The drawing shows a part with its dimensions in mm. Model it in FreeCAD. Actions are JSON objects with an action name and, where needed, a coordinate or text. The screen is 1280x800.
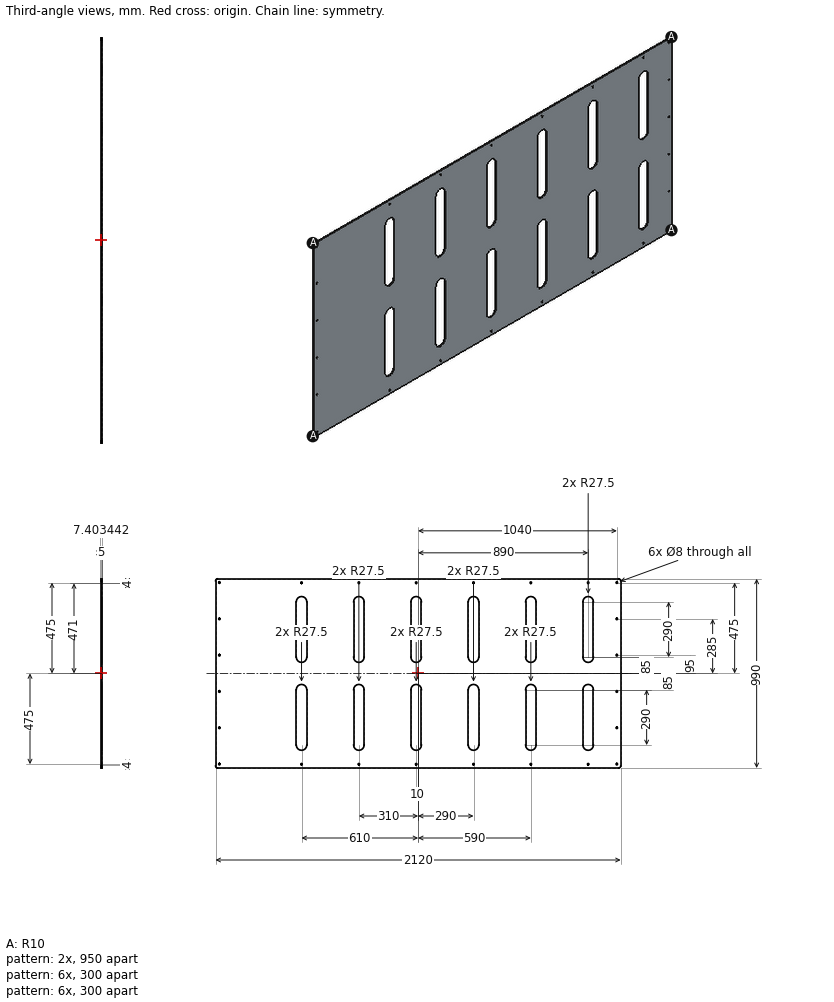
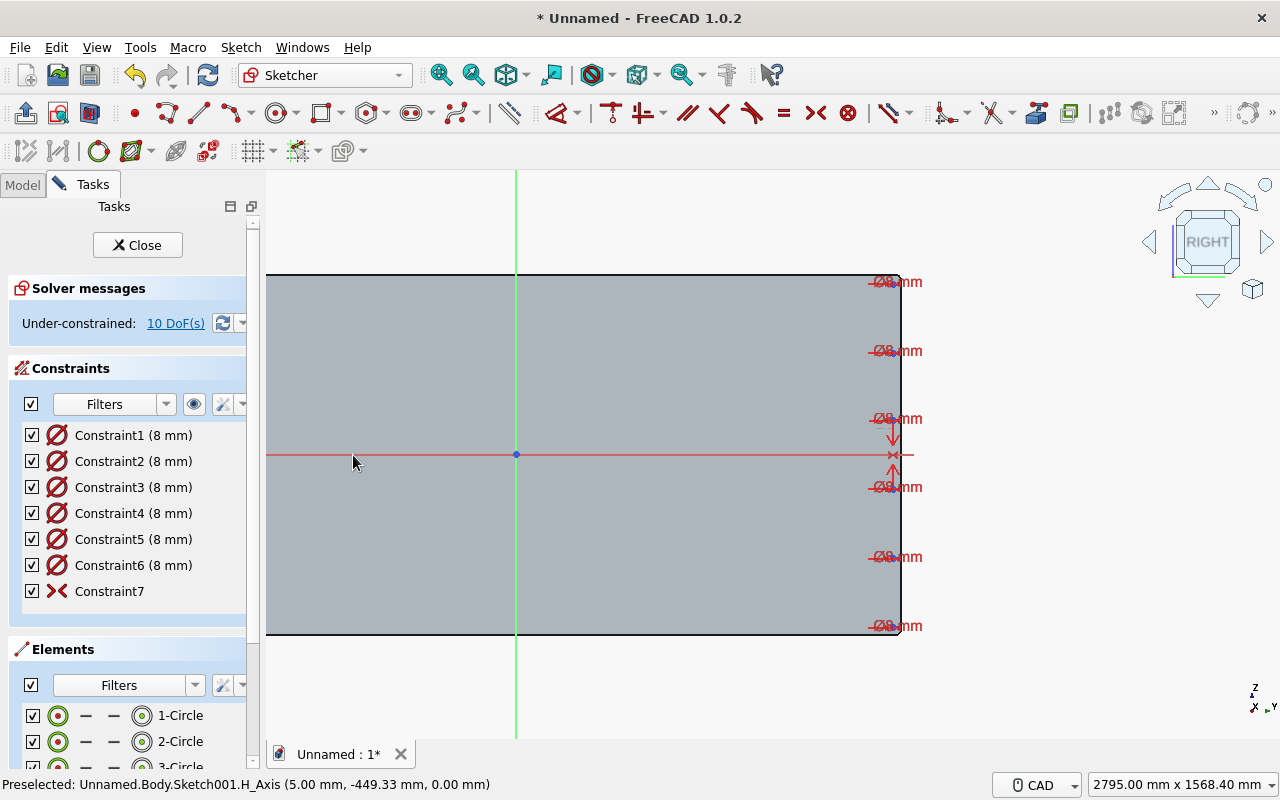
{"action": "left_click", "coordinate": [893, 353]}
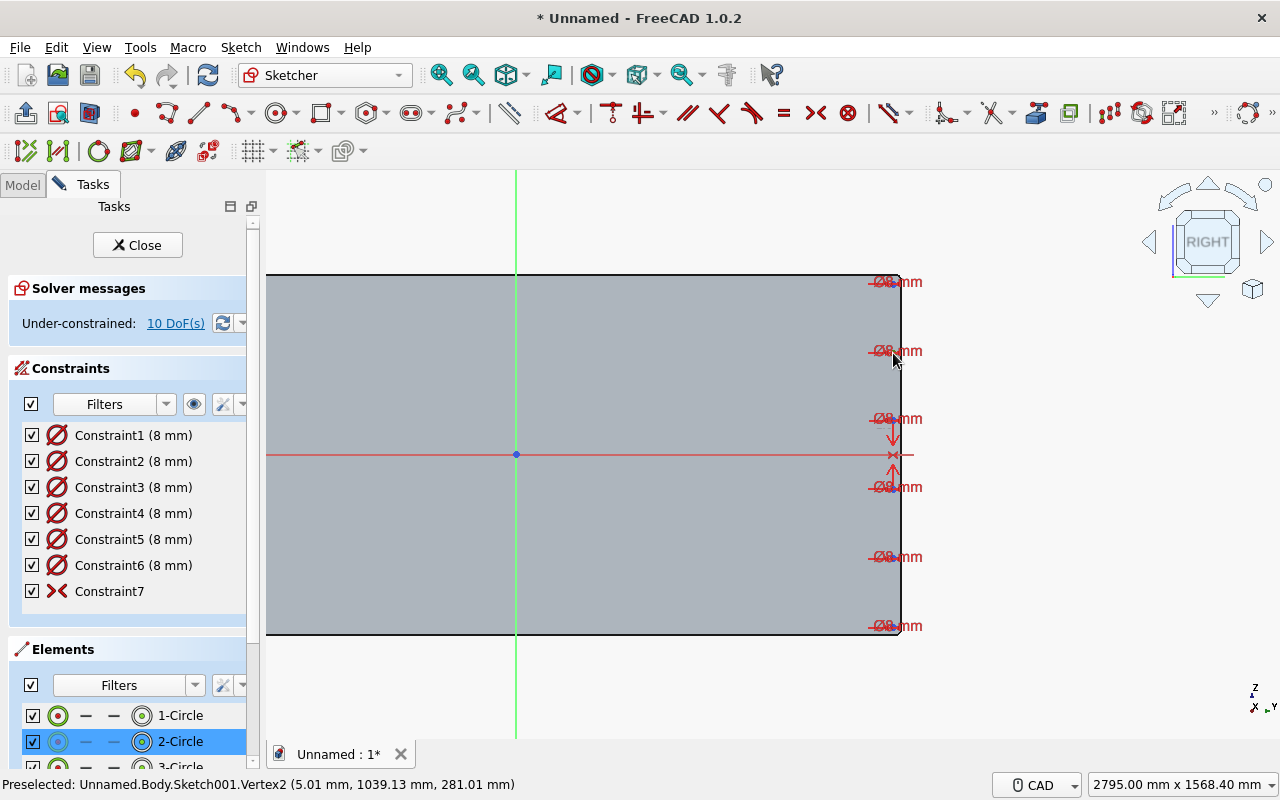
{"action": "left_click", "coordinate": [893, 559]}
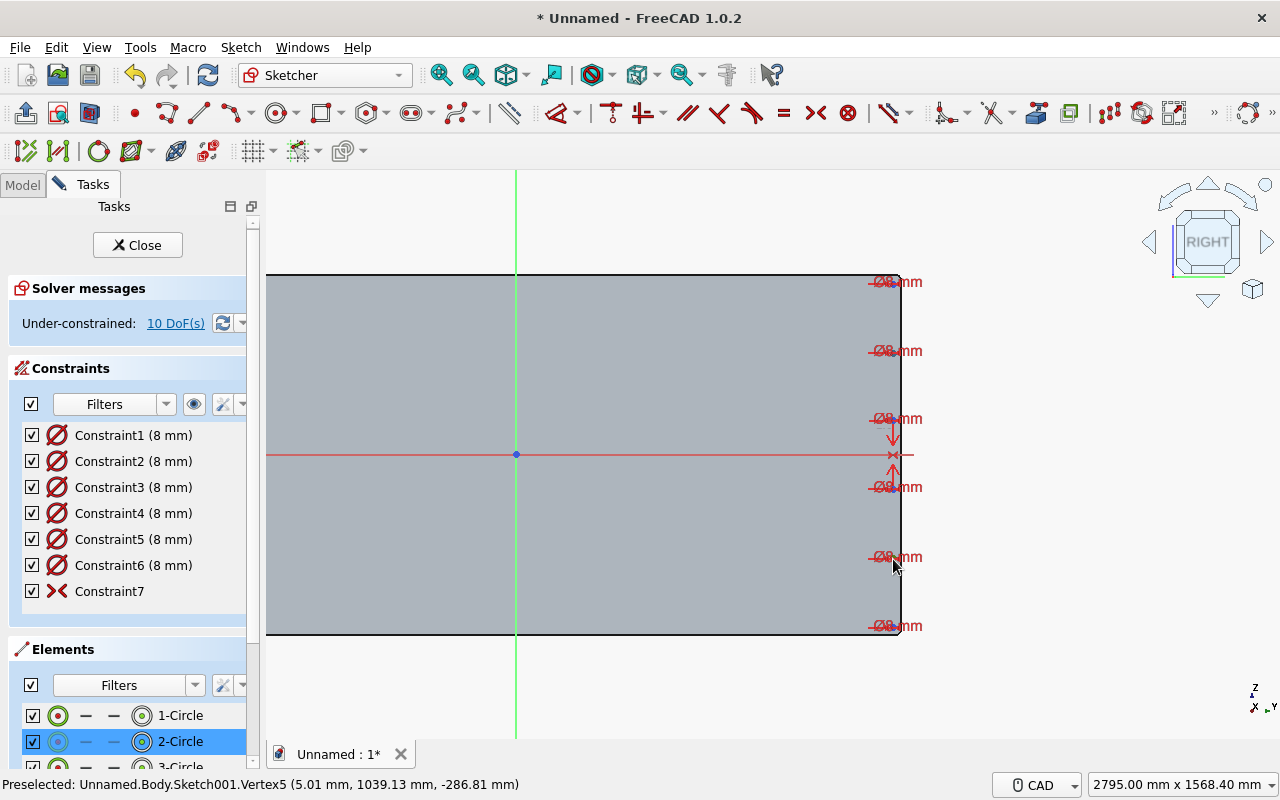
{"action": "left_click", "coordinate": [353, 455]}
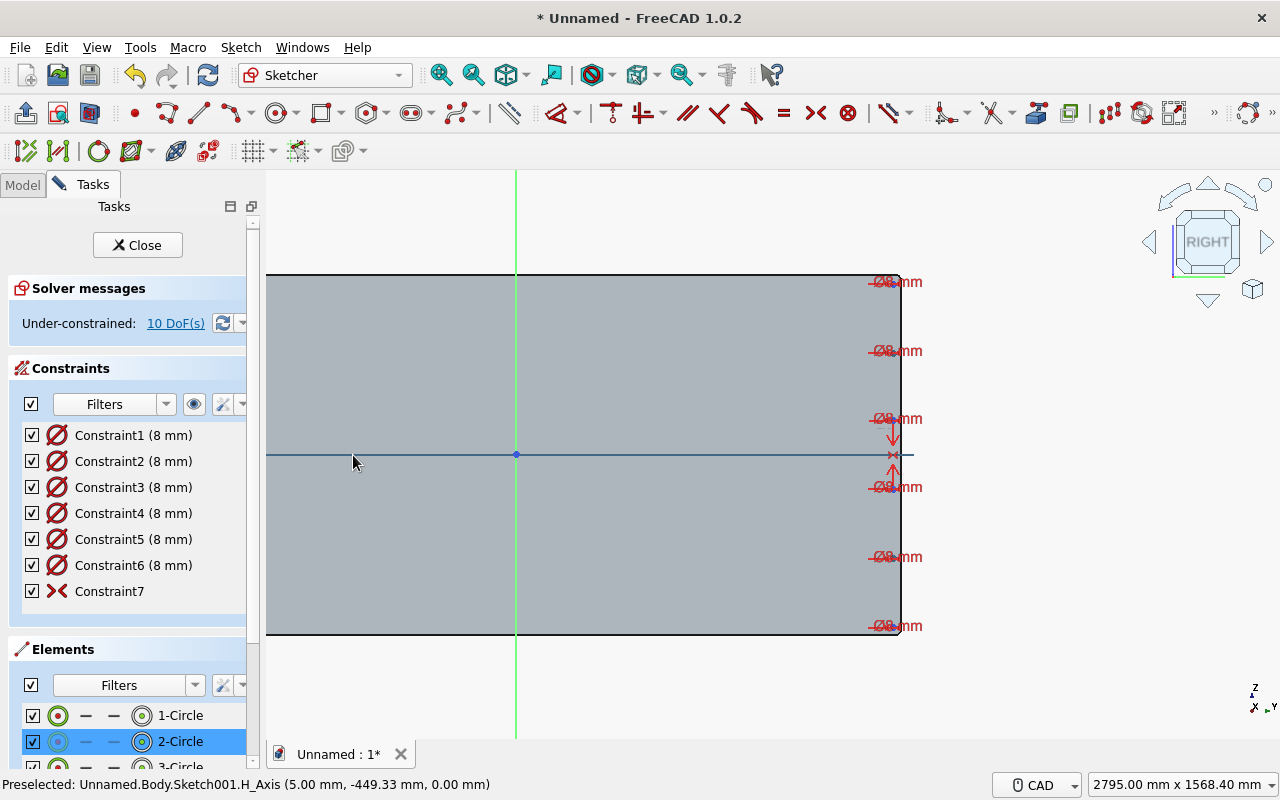
{"action": "left_click", "coordinate": [816, 114]}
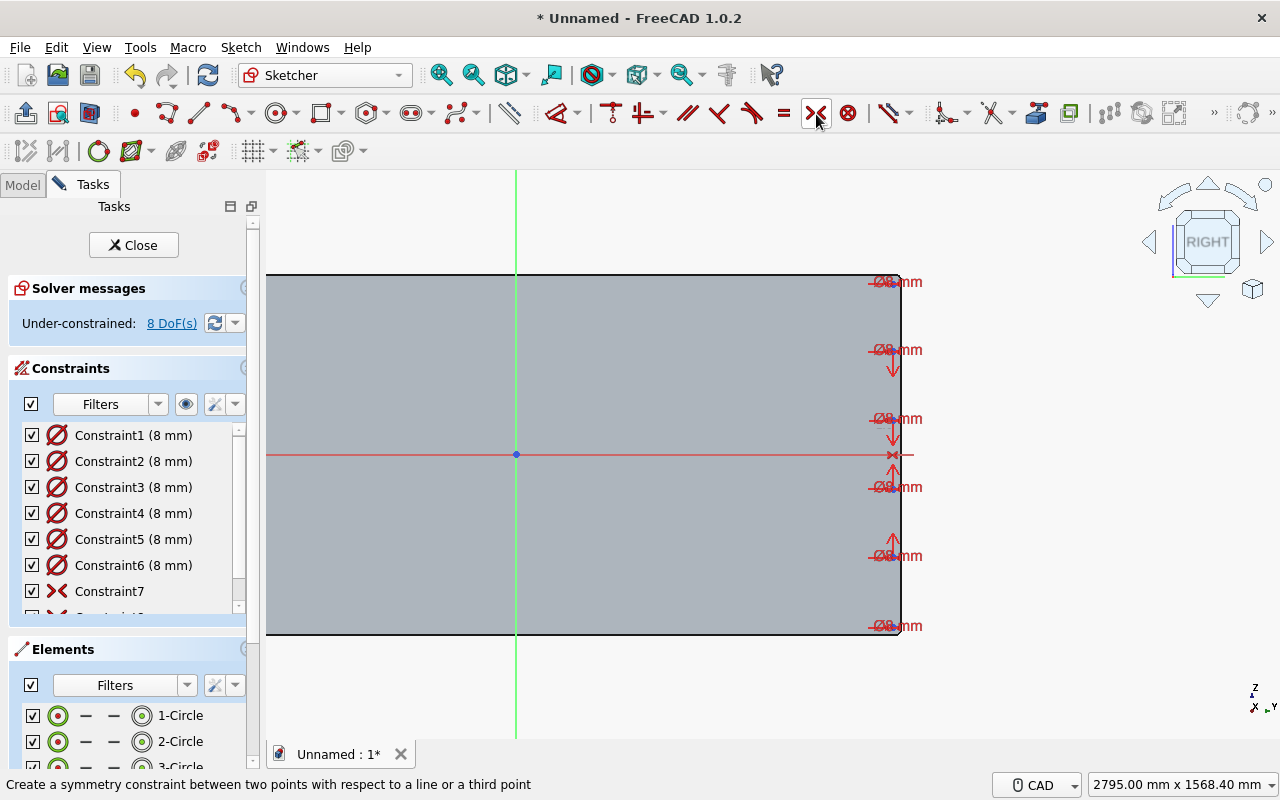
{"action": "left_click", "coordinate": [893, 284]}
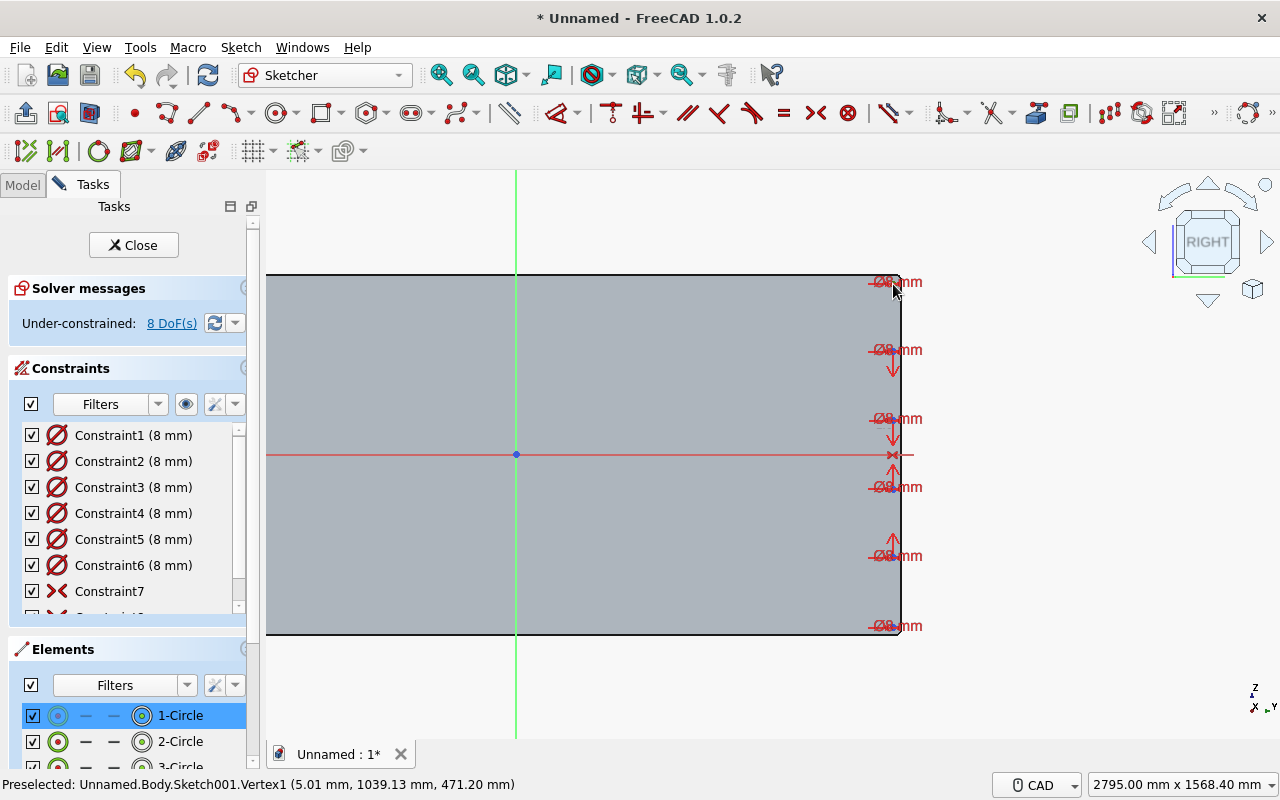
{"action": "left_click", "coordinate": [893, 628]}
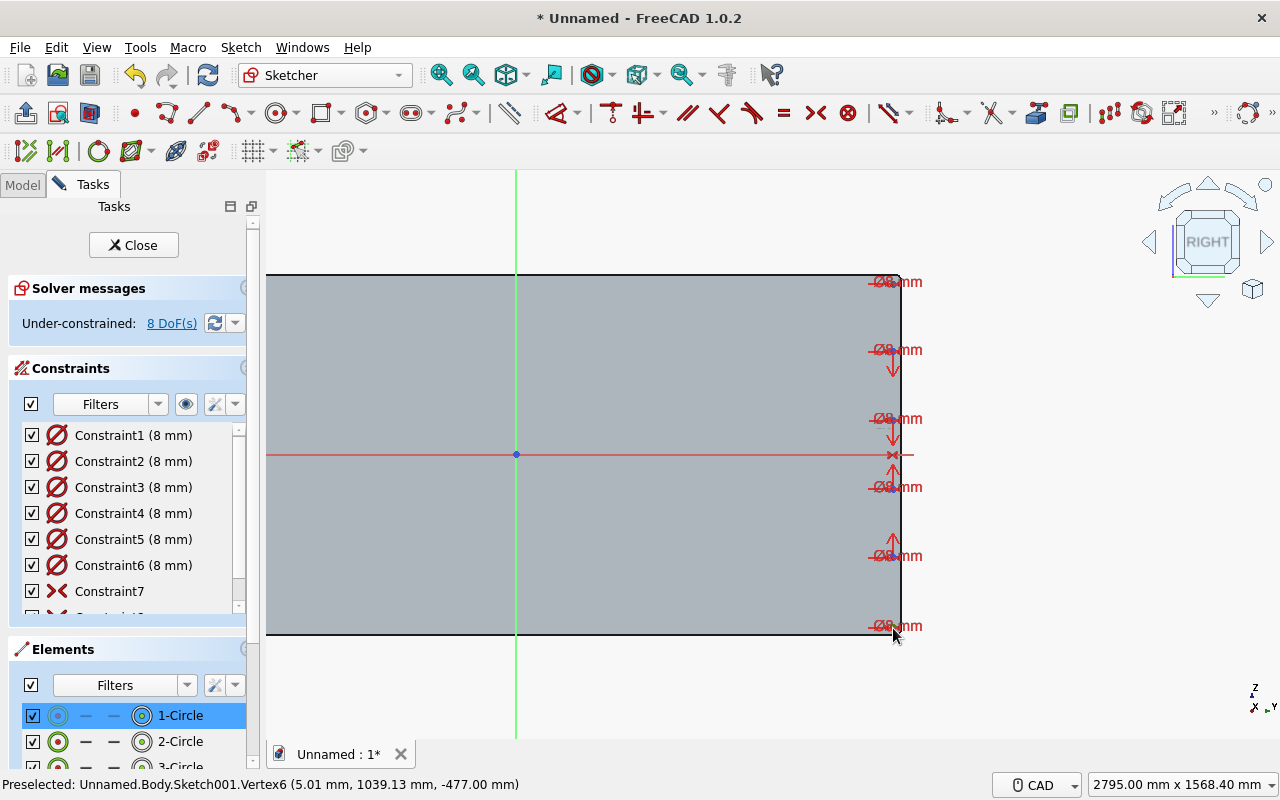
{"action": "left_click", "coordinate": [353, 455]}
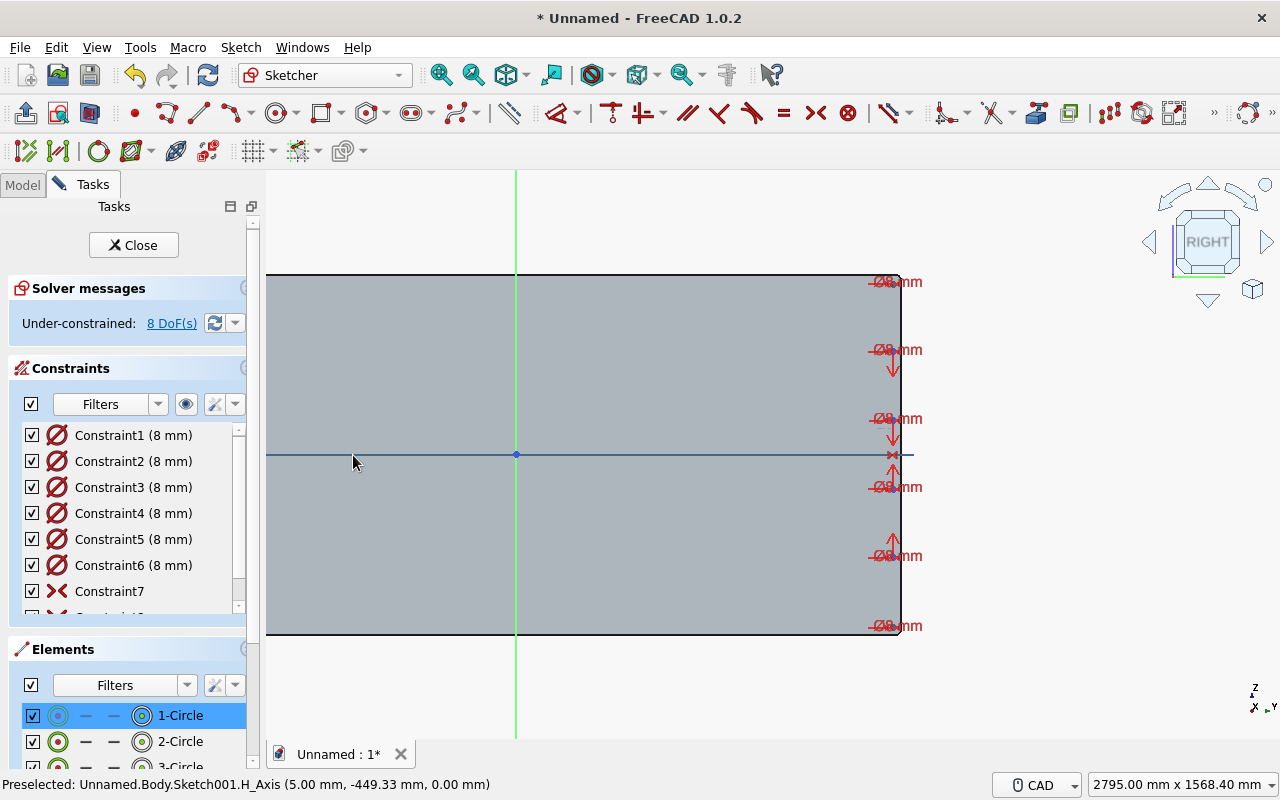
{"action": "left_click", "coordinate": [816, 114]}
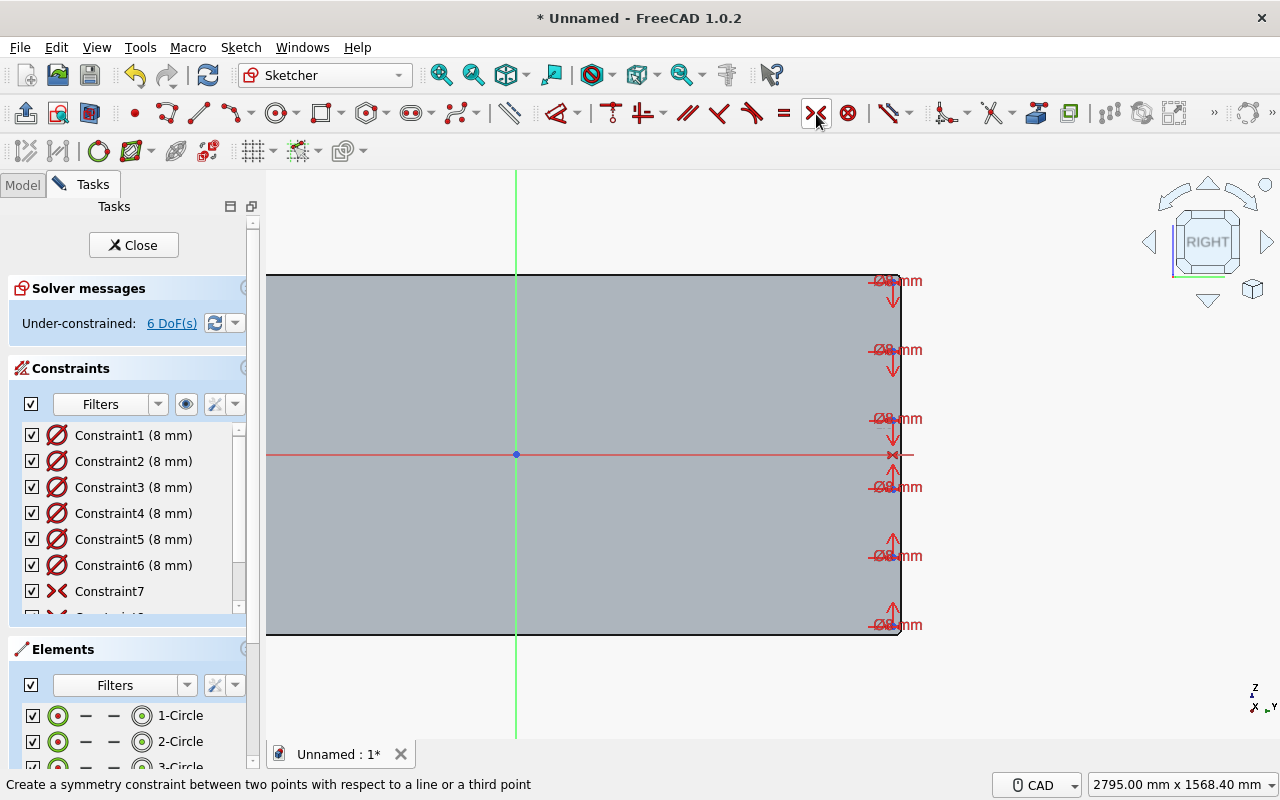
{"action": "left_click", "coordinate": [556, 114]}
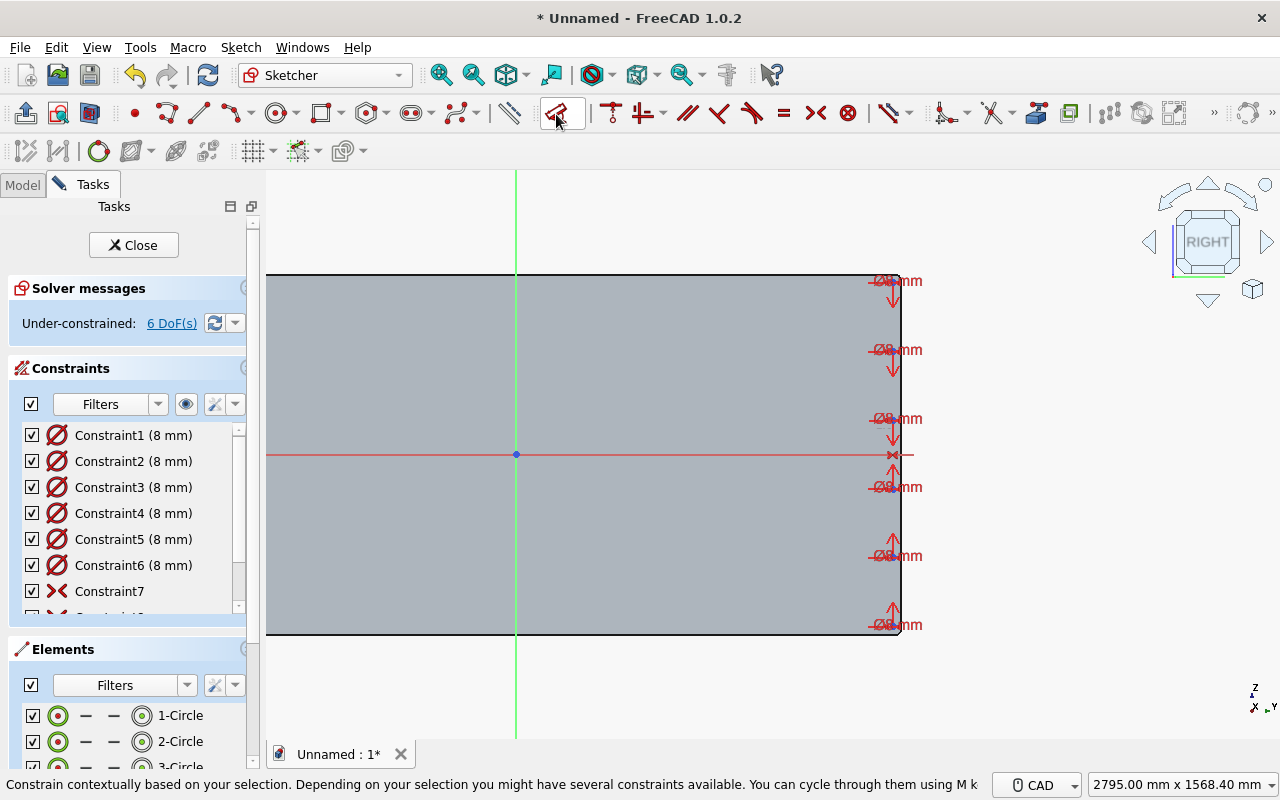
{"action": "left_click", "coordinate": [893, 421]}
{"action": "left_click", "coordinate": [482, 438]}